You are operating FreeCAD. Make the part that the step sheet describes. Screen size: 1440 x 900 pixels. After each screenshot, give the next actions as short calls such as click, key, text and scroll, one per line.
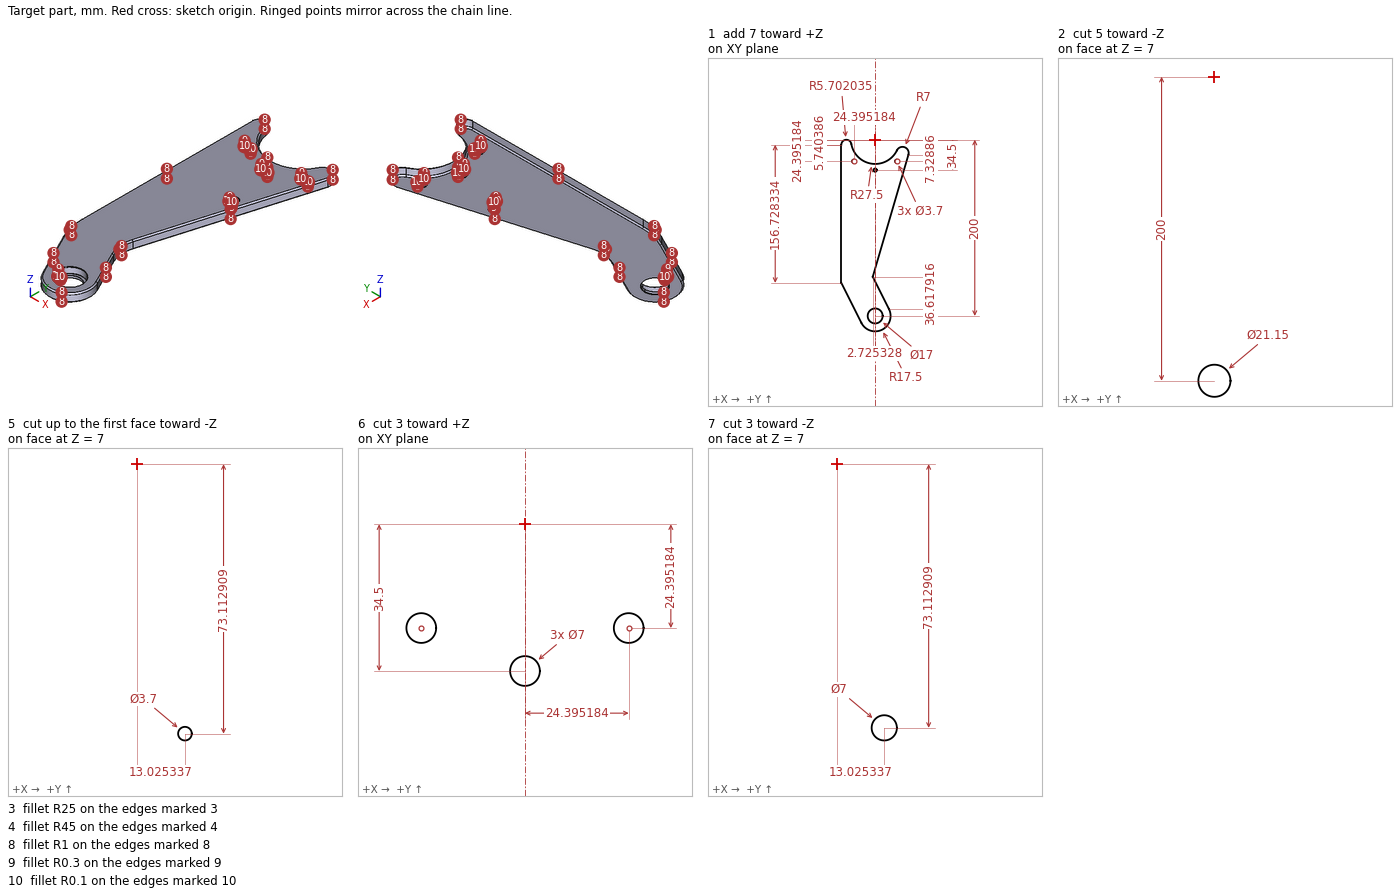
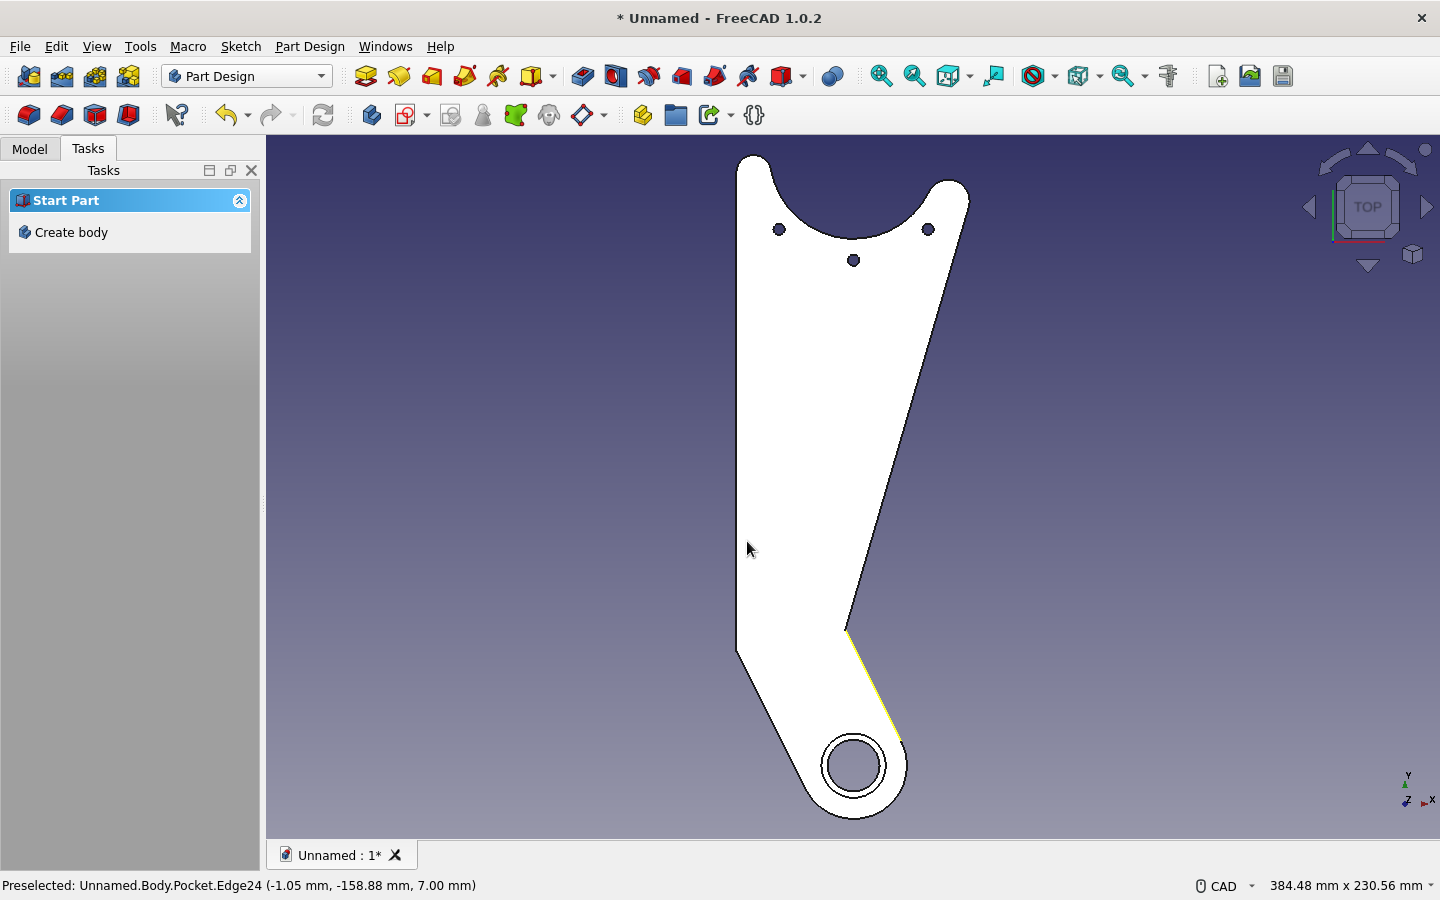
scroll(845, 629, up, 4)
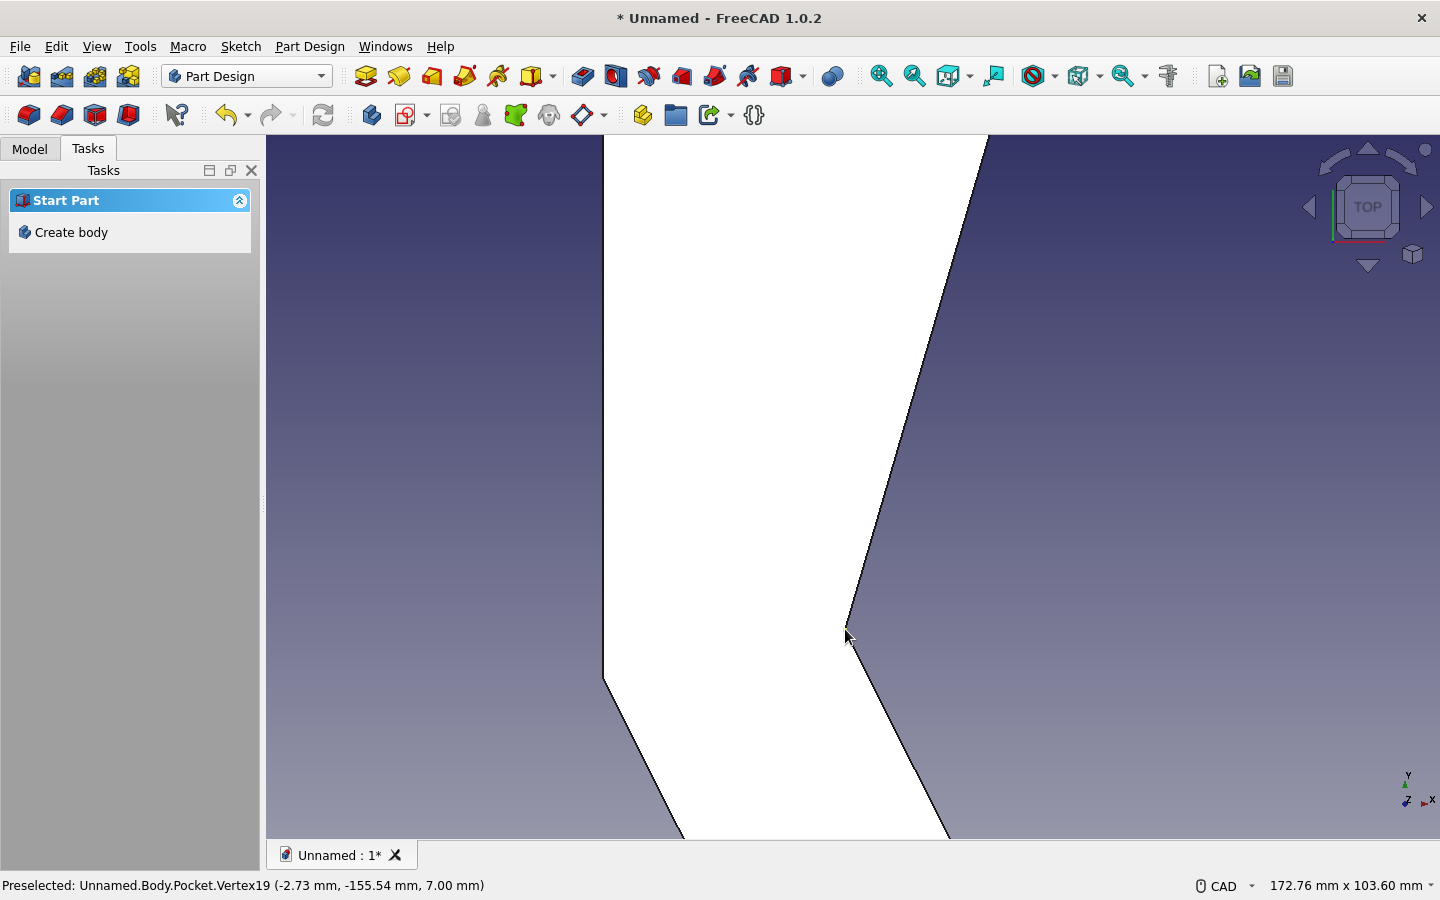
click(882, 76)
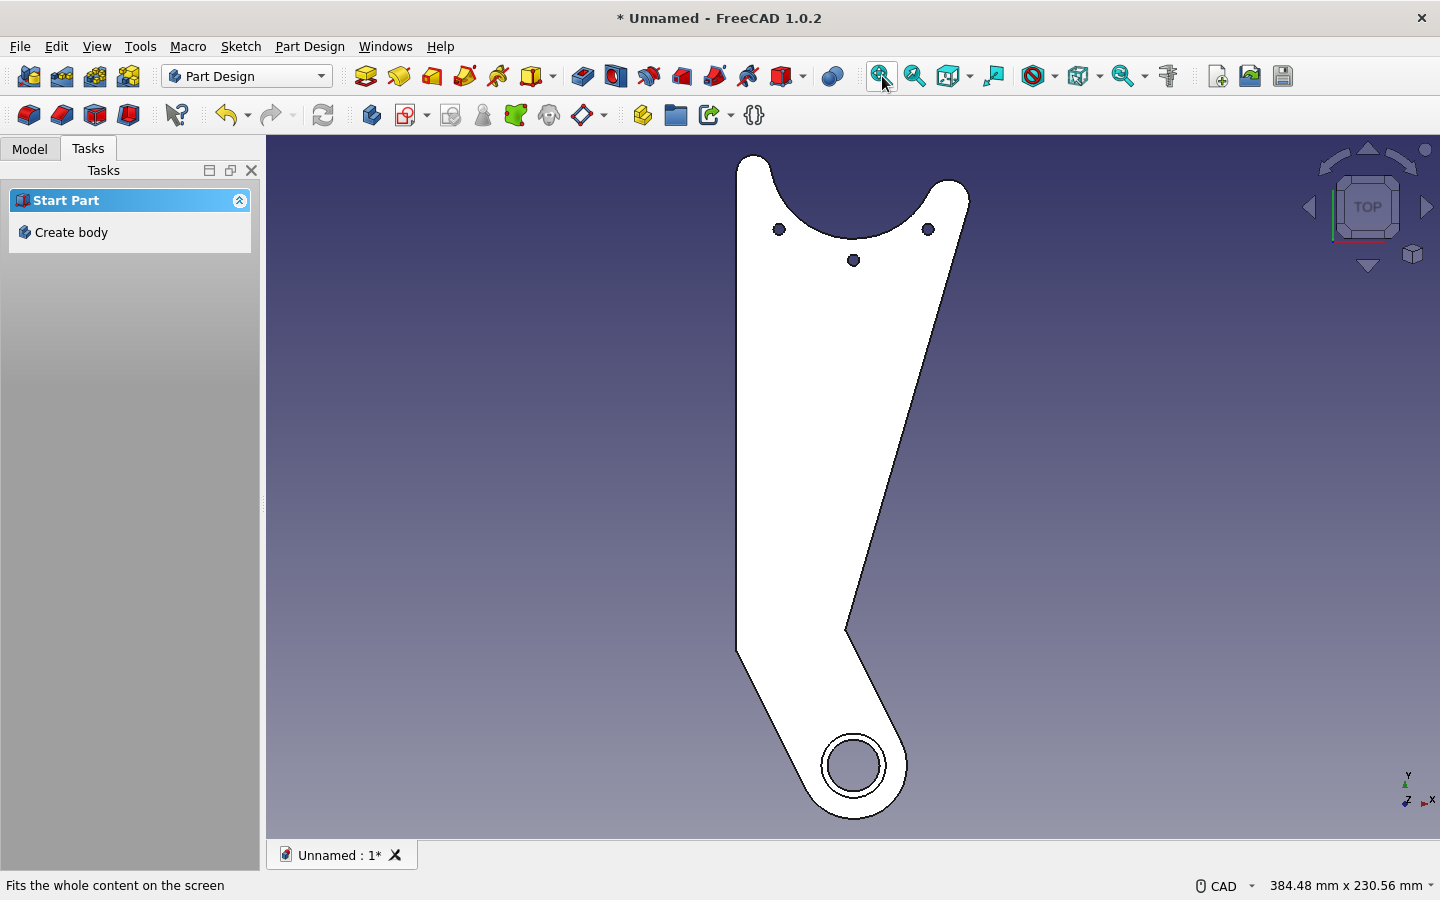
key(1)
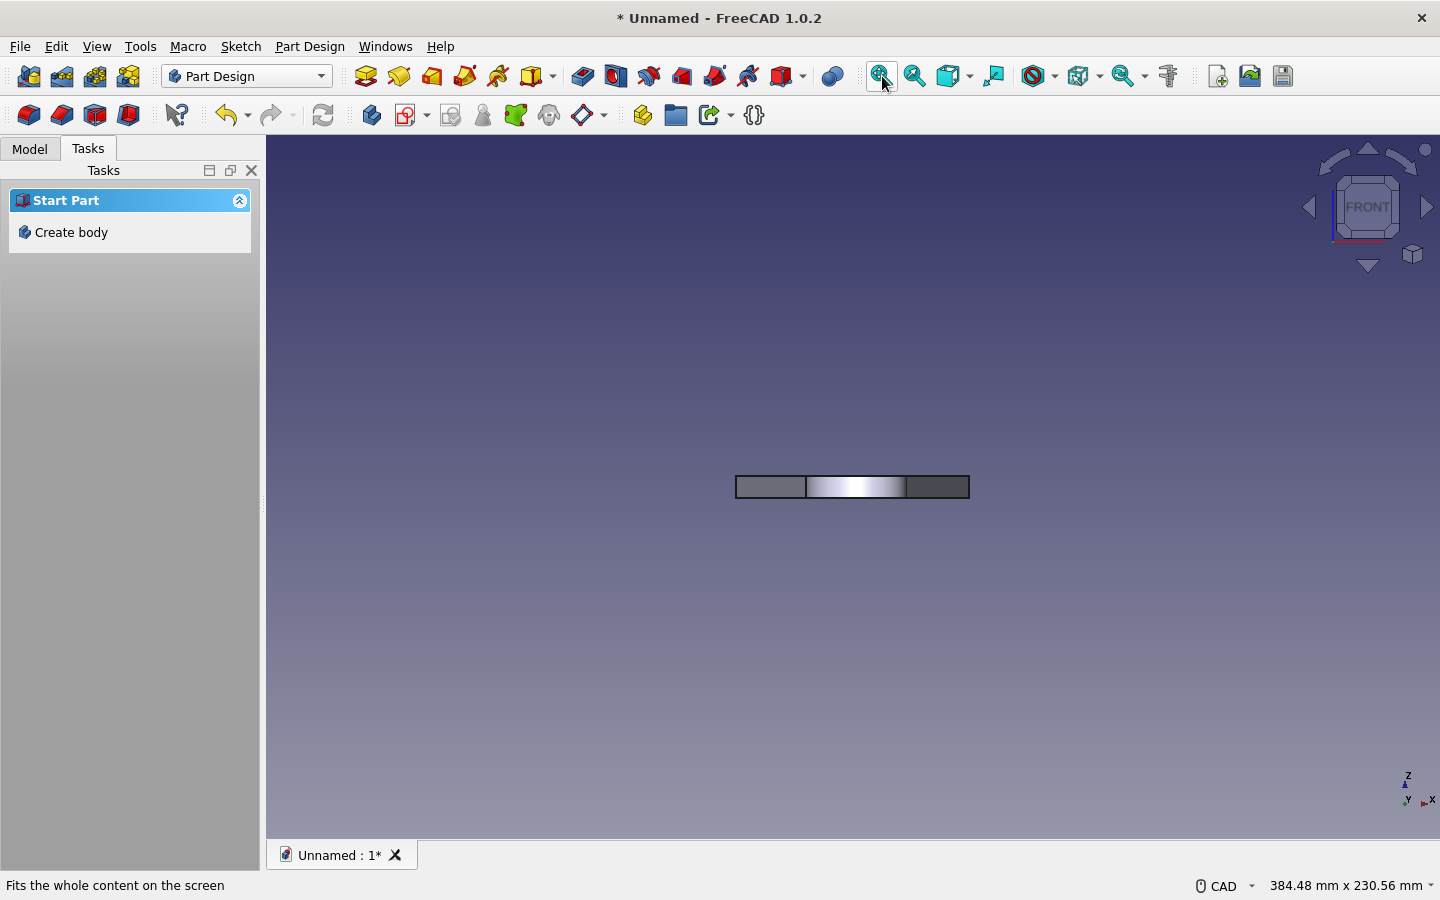
key(v)
key(f)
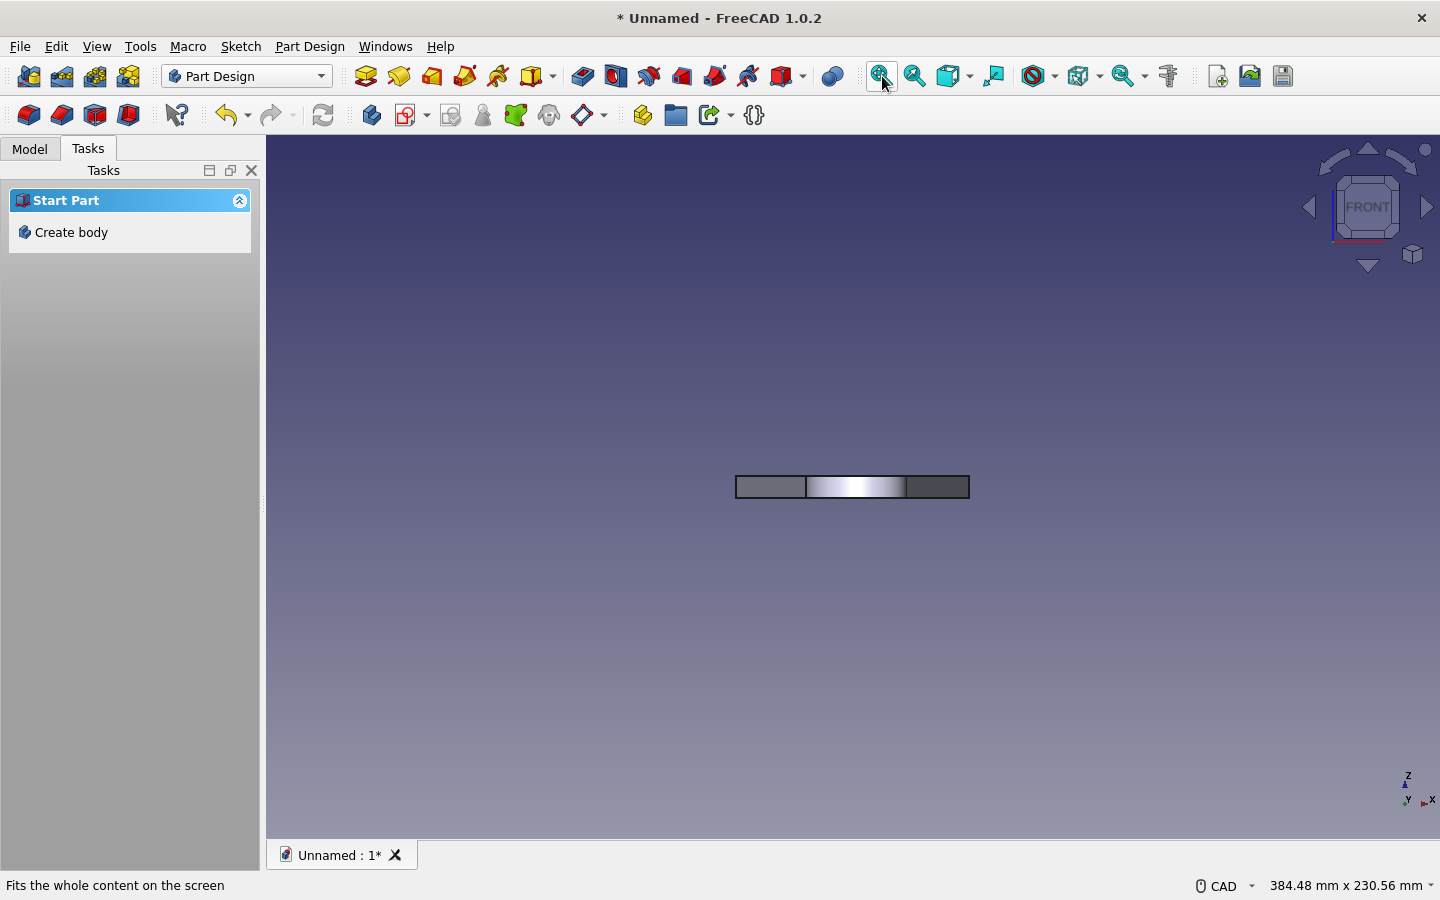
scroll(845, 486, up, 4)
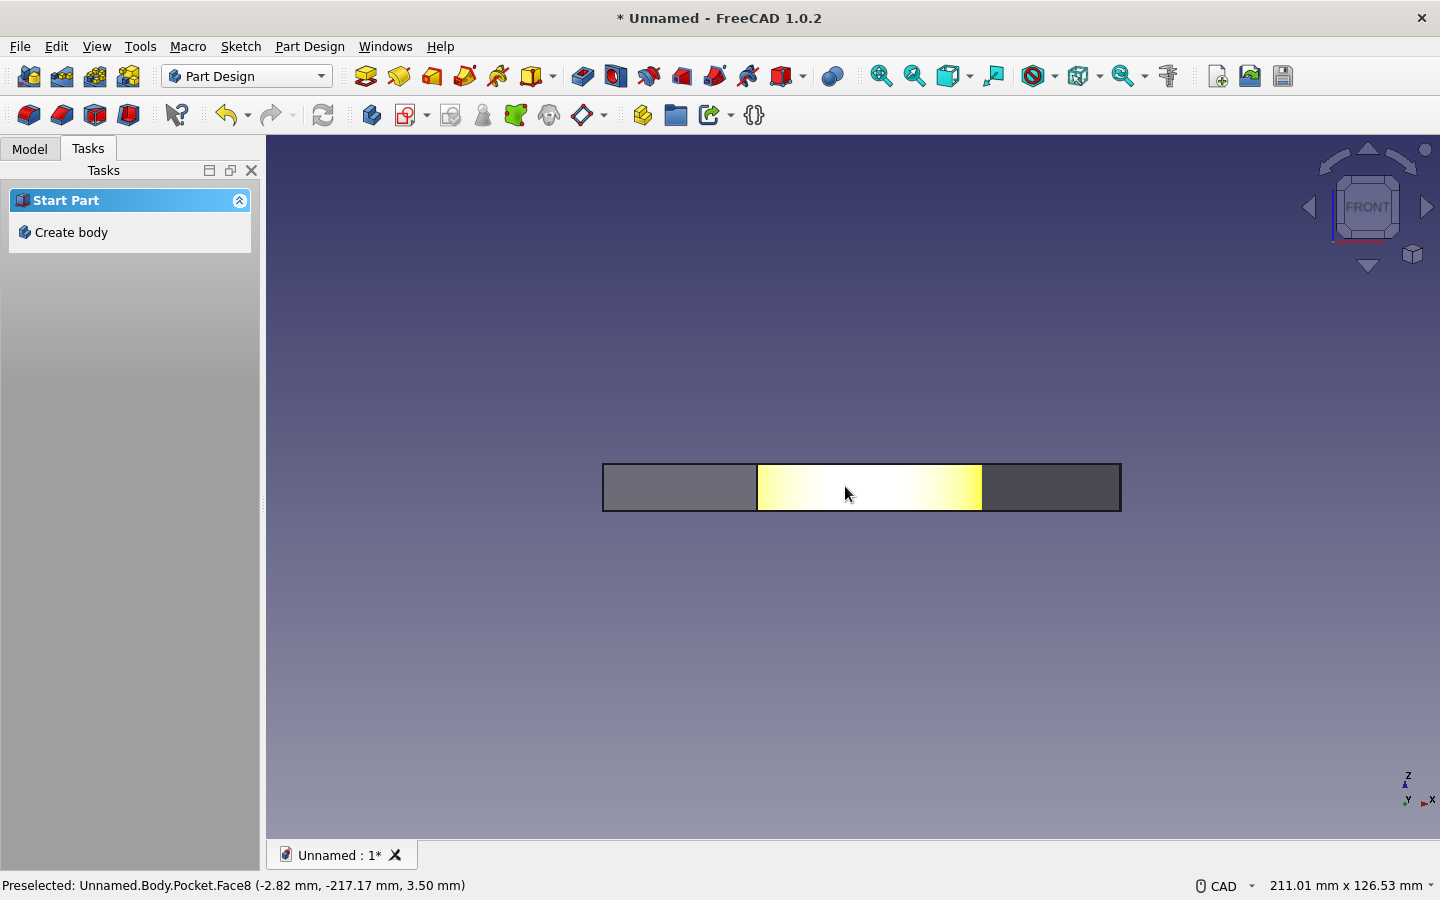
click(882, 76)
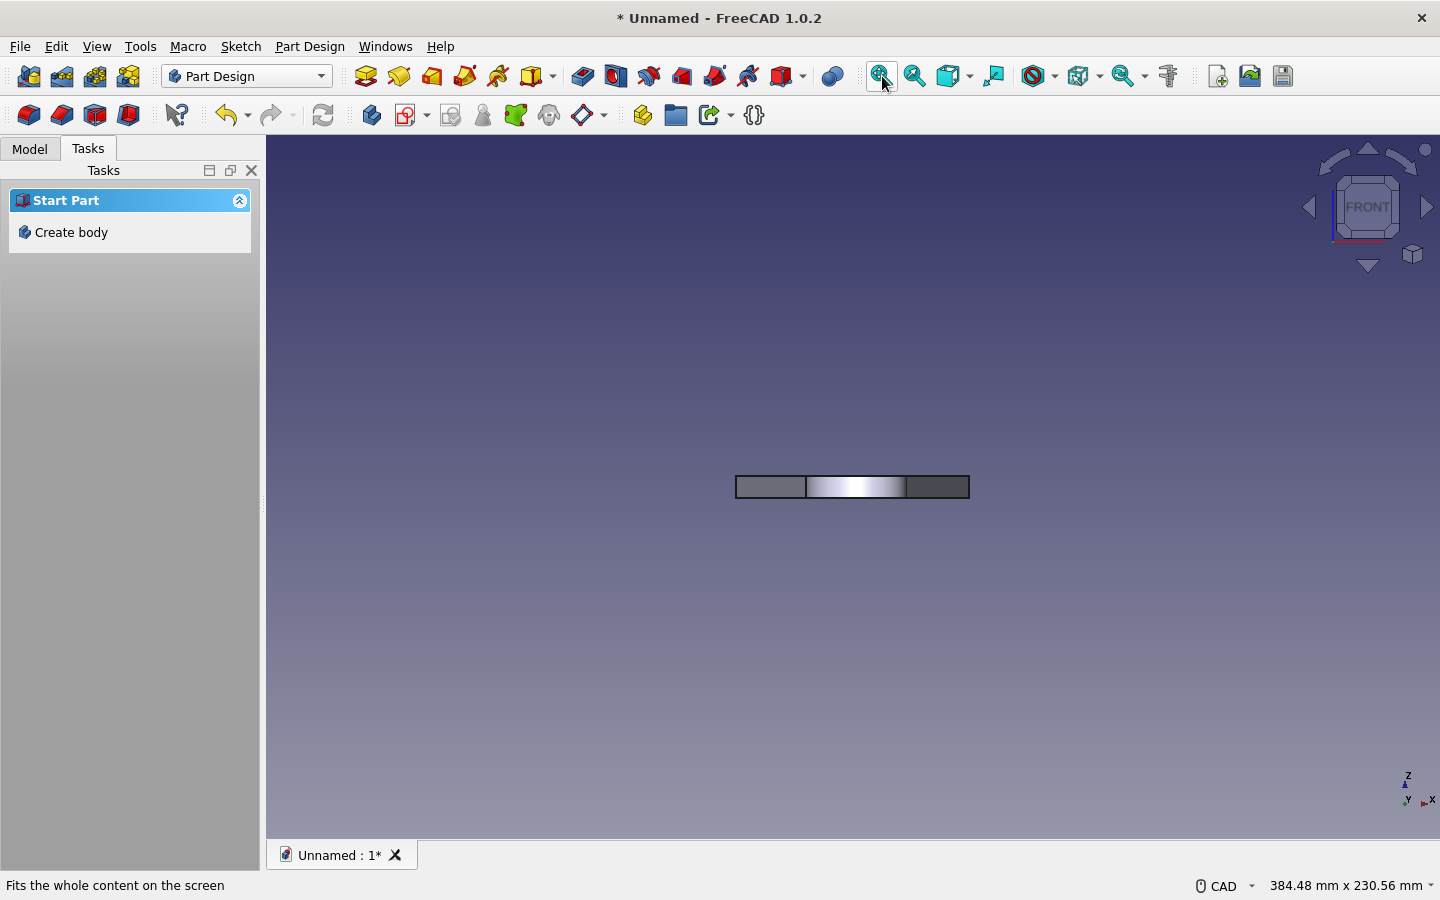
key(3)